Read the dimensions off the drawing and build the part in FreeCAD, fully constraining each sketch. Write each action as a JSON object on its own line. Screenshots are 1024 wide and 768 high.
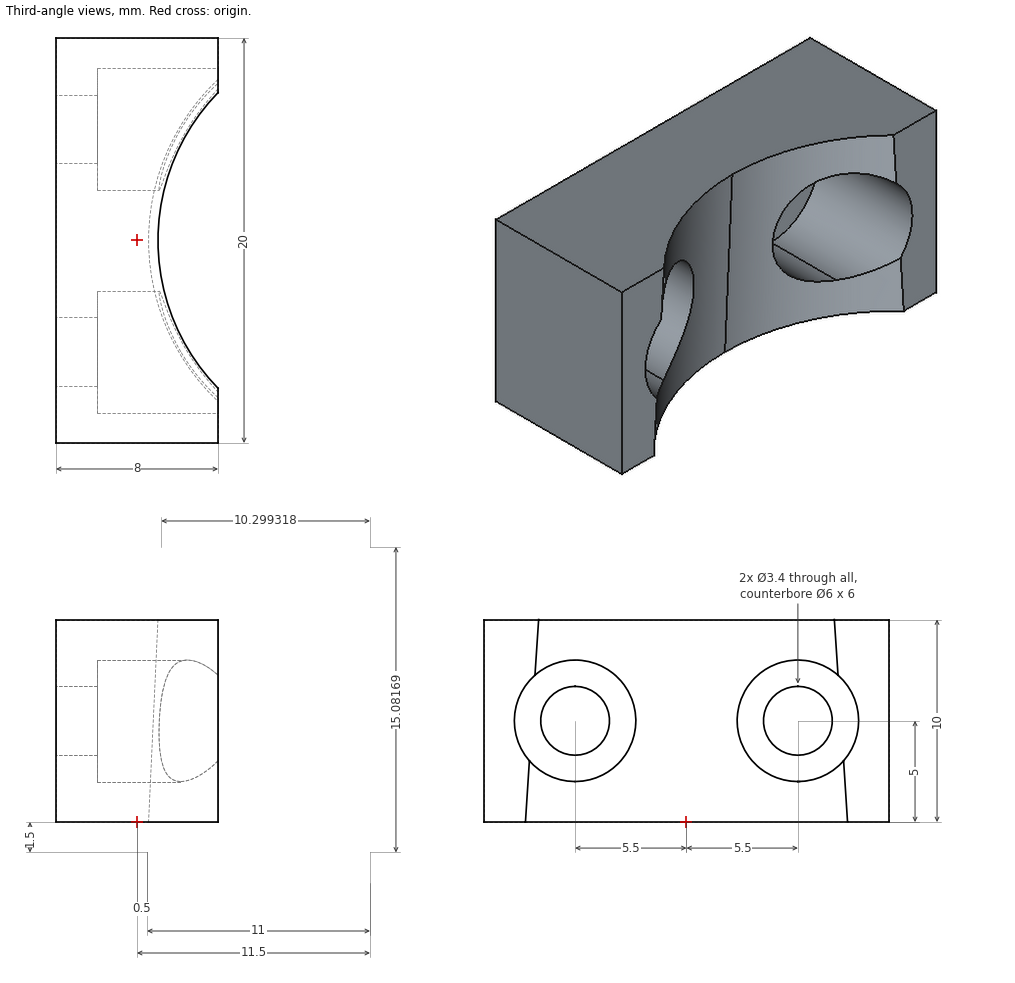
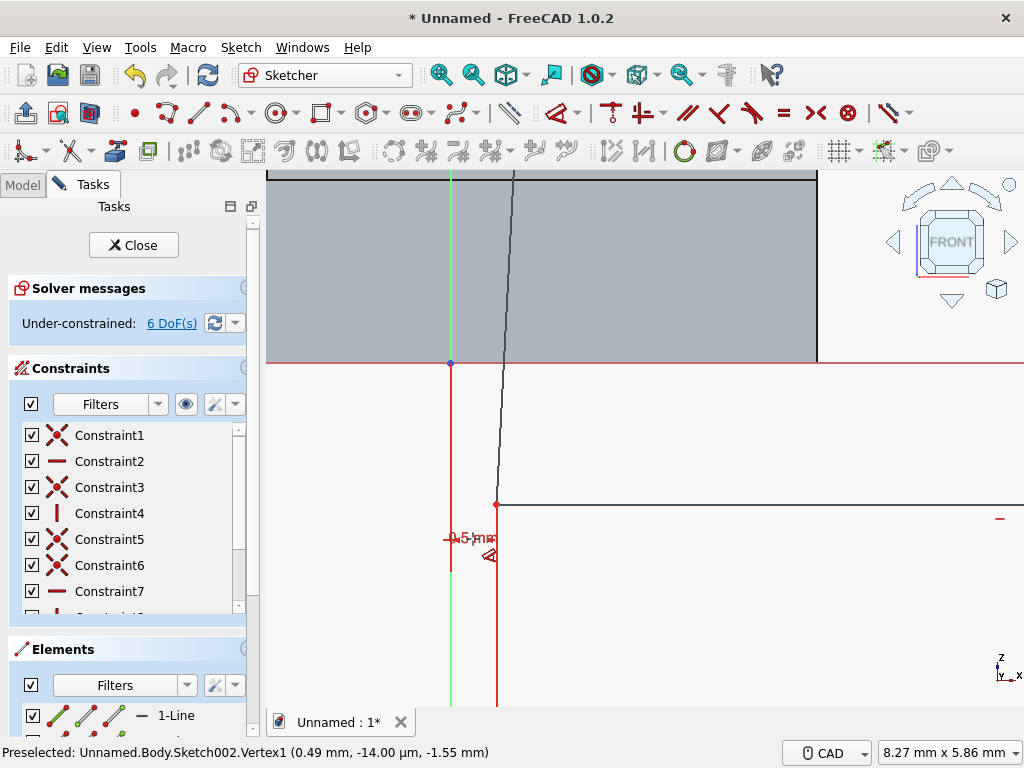
{"action": "scroll", "coordinate": [497, 508], "scroll_direction": "down", "scroll_amount": 9}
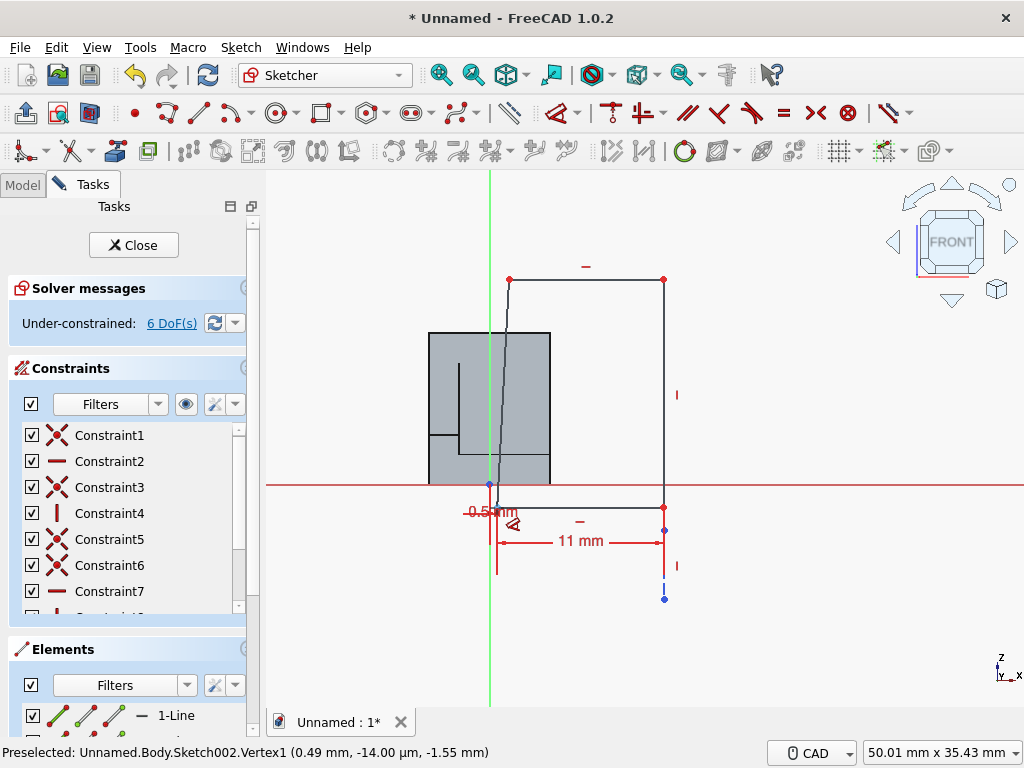
{"action": "scroll", "coordinate": [497, 508], "scroll_direction": "up", "scroll_amount": 3}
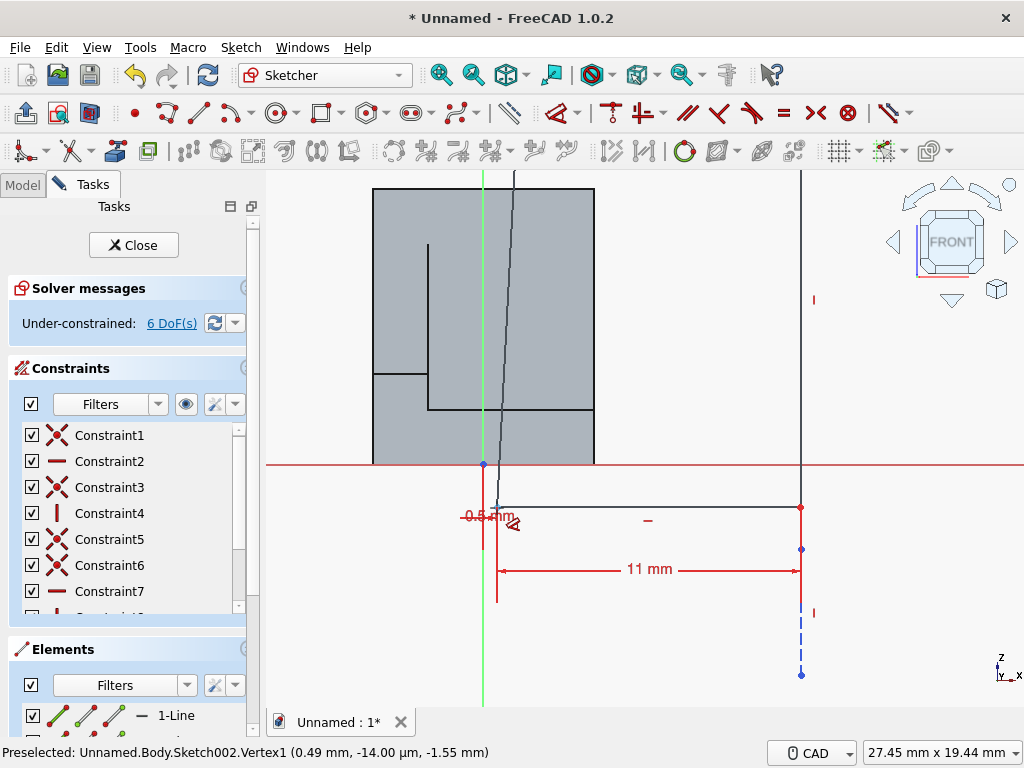
{"action": "left_click", "coordinate": [497, 507]}
{"action": "left_click", "coordinate": [449, 486]}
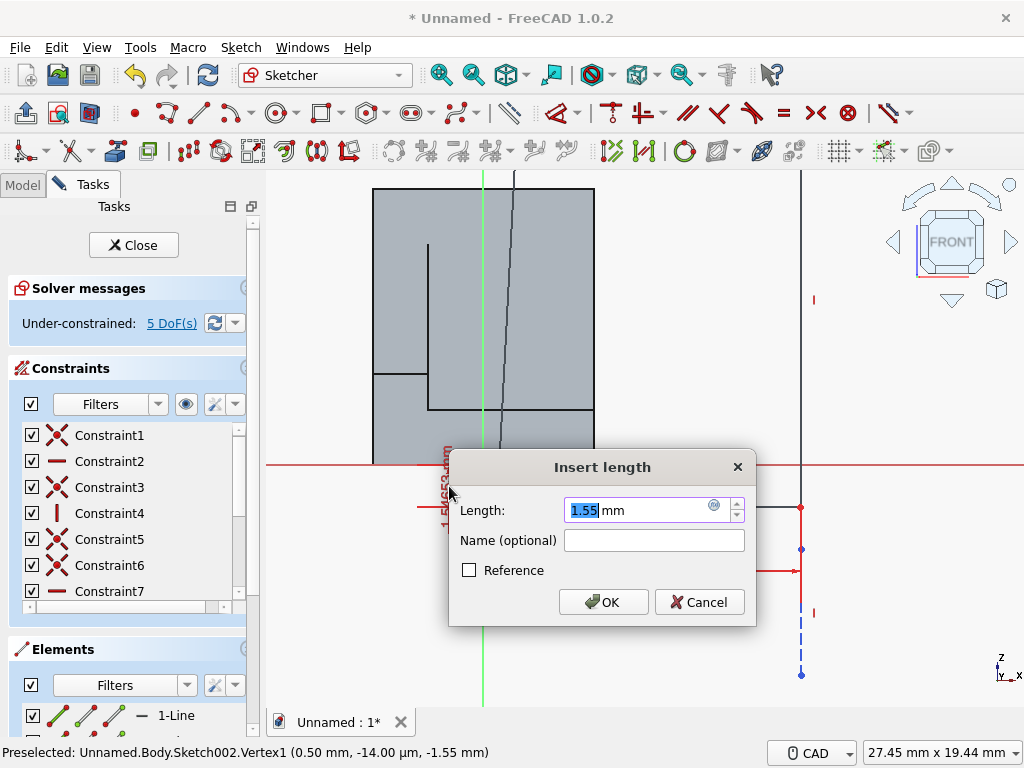
{"action": "type", "text": "1.5"}
{"action": "key", "text": "Return"}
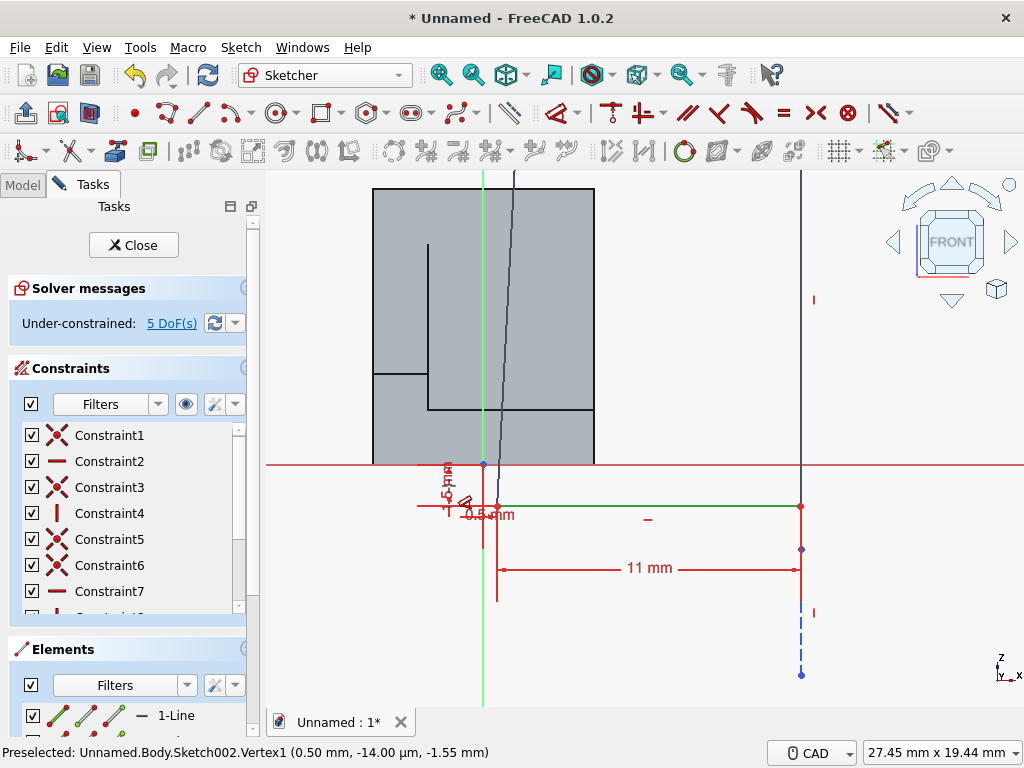
{"action": "left_click", "coordinate": [801, 549]}
{"action": "left_click", "coordinate": [569, 583]}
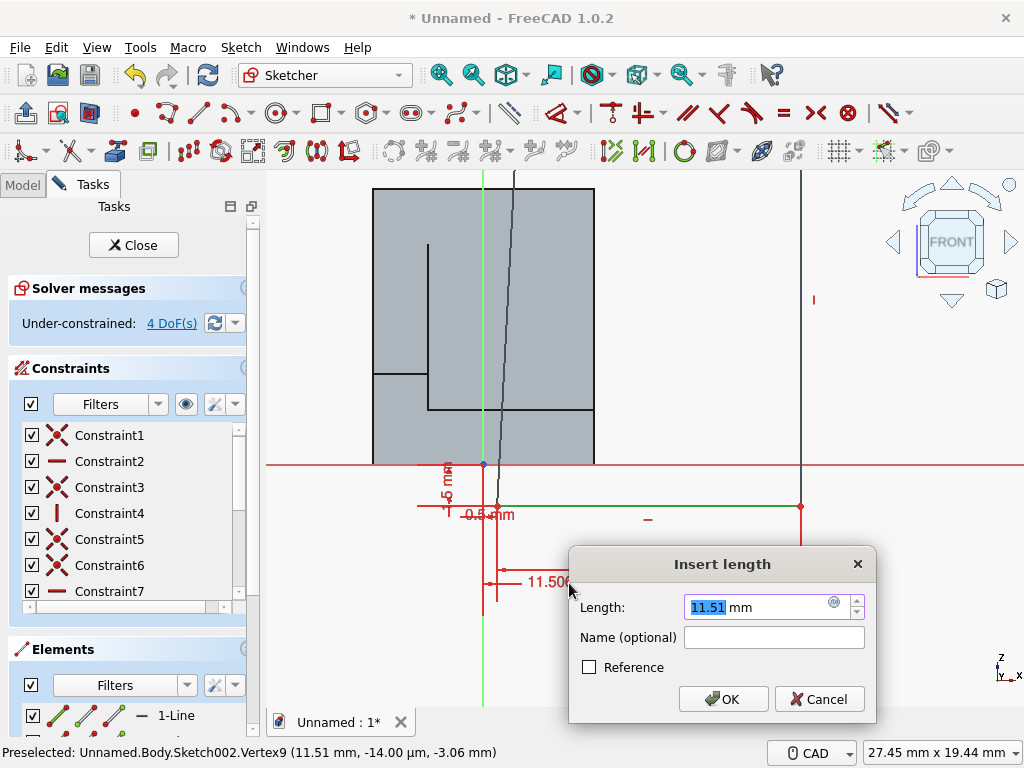
{"action": "type", "text": "11.5"}
{"action": "key", "text": "Return"}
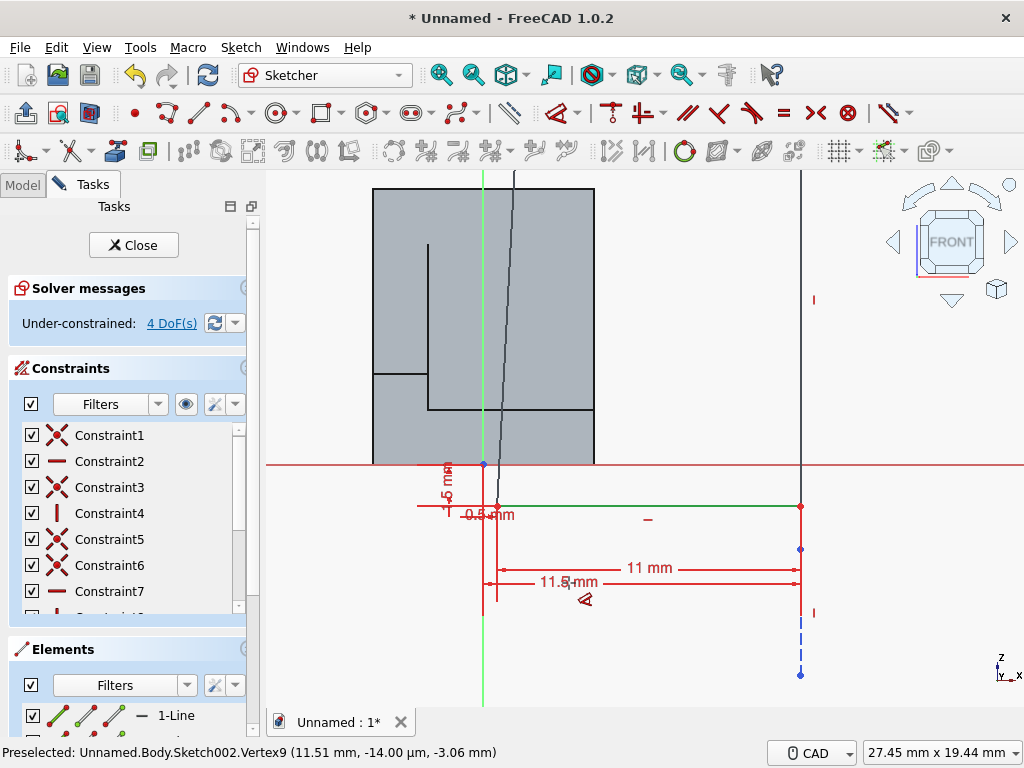
{"action": "left_click", "coordinate": [801, 216]}
{"action": "left_click", "coordinate": [835, 352]}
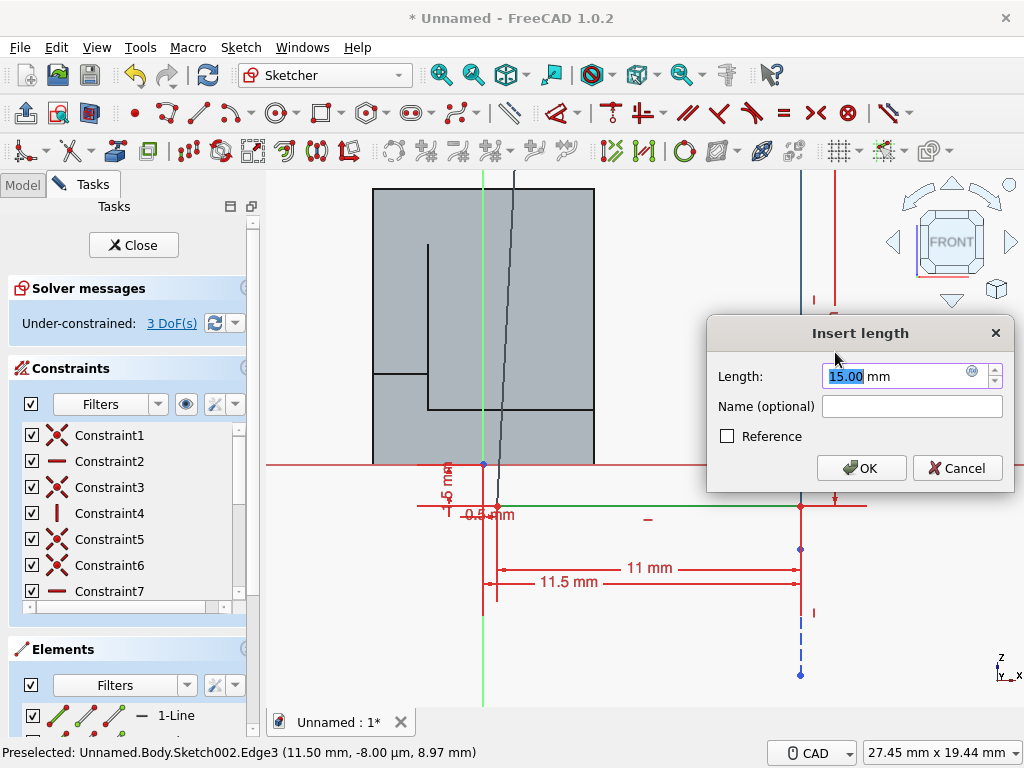
{"action": "type", "text": "15.08169"}
{"action": "key", "text": "Return"}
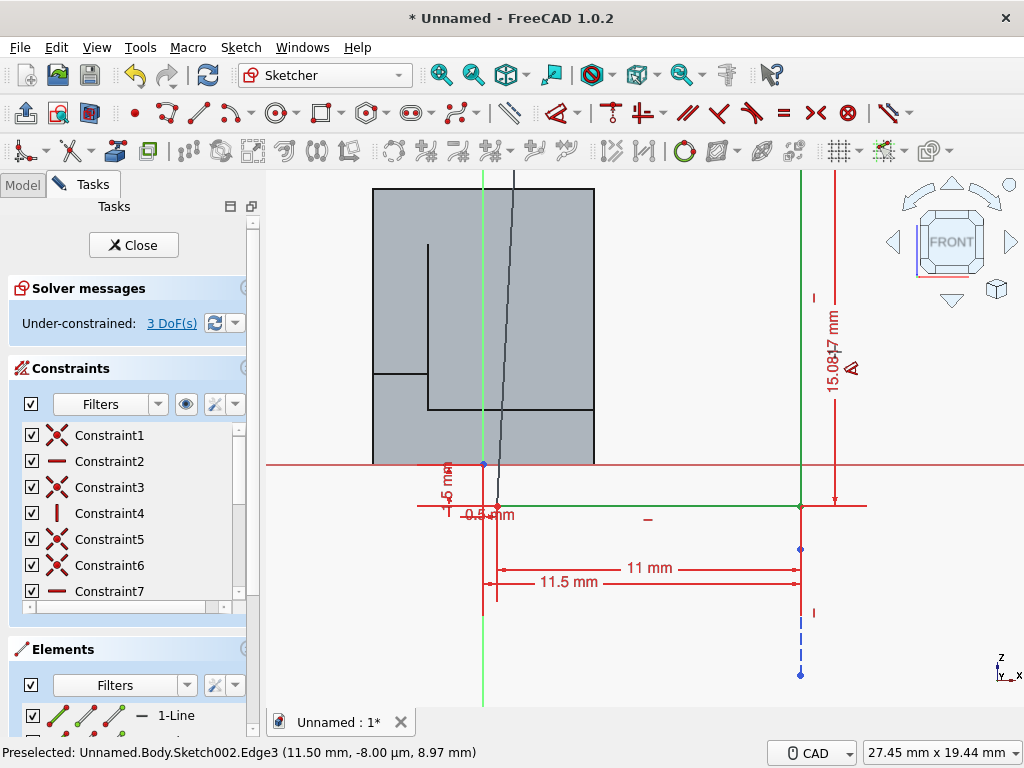
{"action": "scroll", "coordinate": [497, 508], "scroll_direction": "down", "scroll_amount": 3}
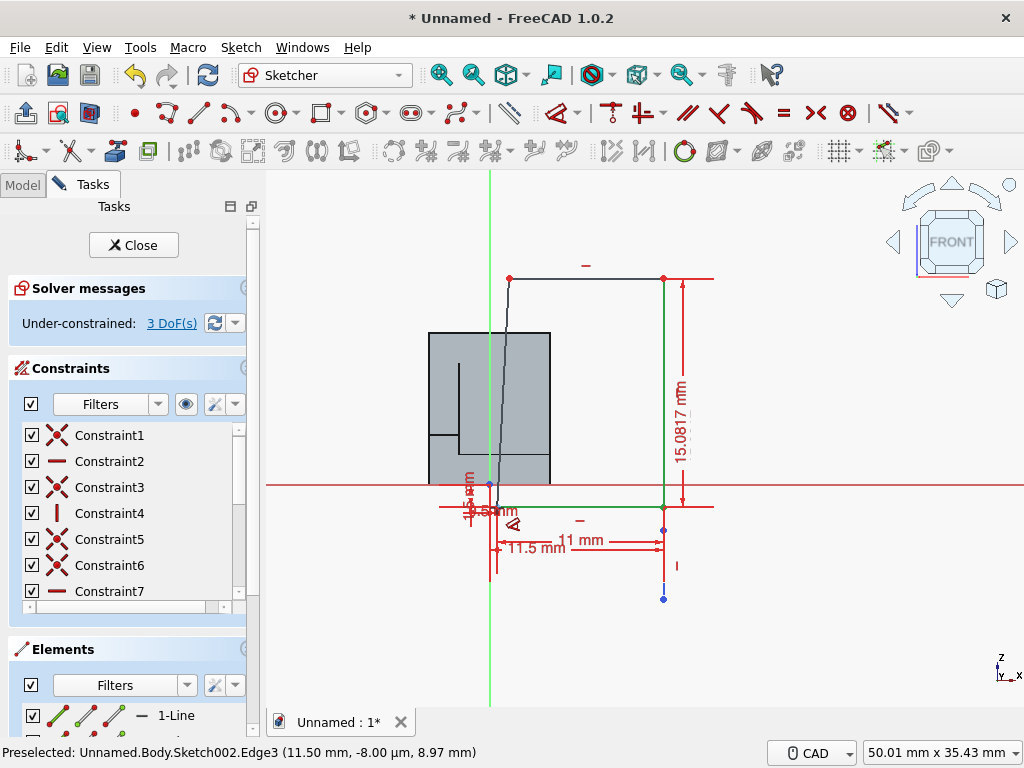
{"action": "left_click", "coordinate": [555, 279]}
{"action": "left_click", "coordinate": [586, 245]}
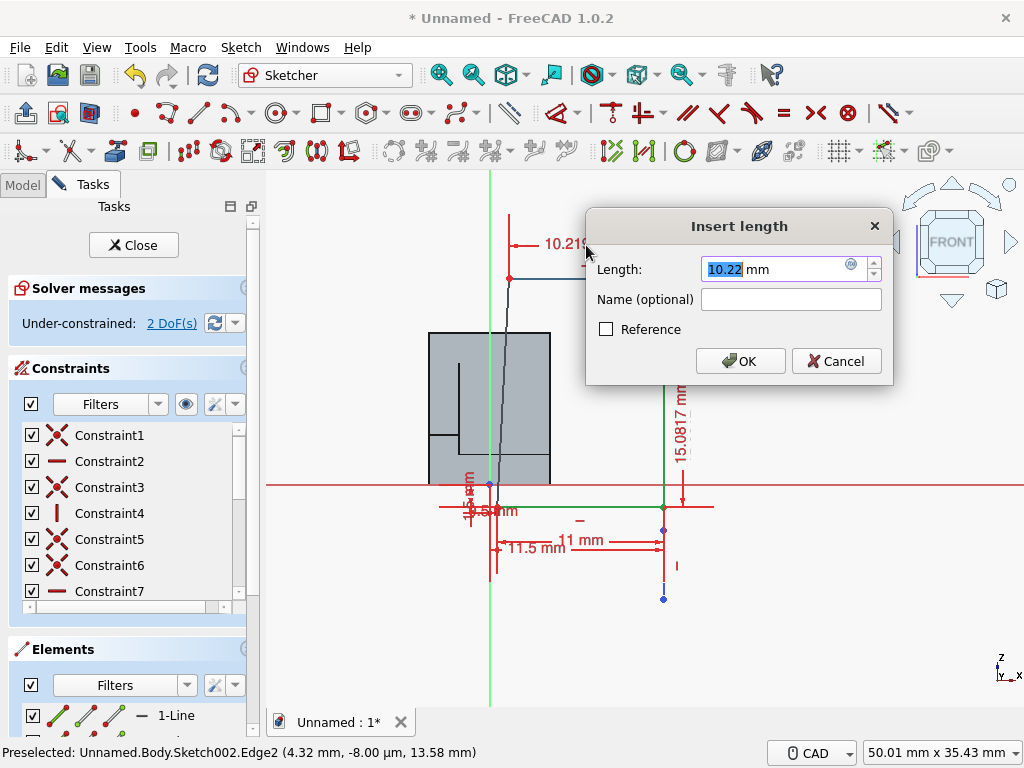
{"action": "type", "text": "10.299318"}
{"action": "key", "text": "Return"}
{"action": "key", "text": "Escape"}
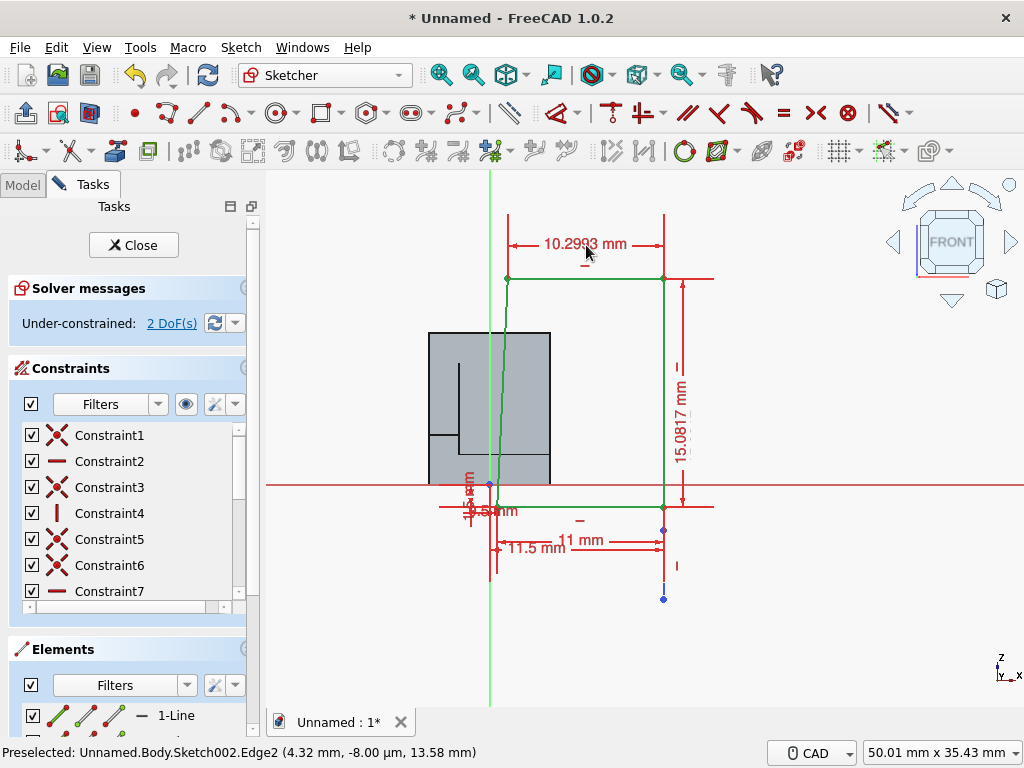
{"action": "left_click", "coordinate": [134, 245]}